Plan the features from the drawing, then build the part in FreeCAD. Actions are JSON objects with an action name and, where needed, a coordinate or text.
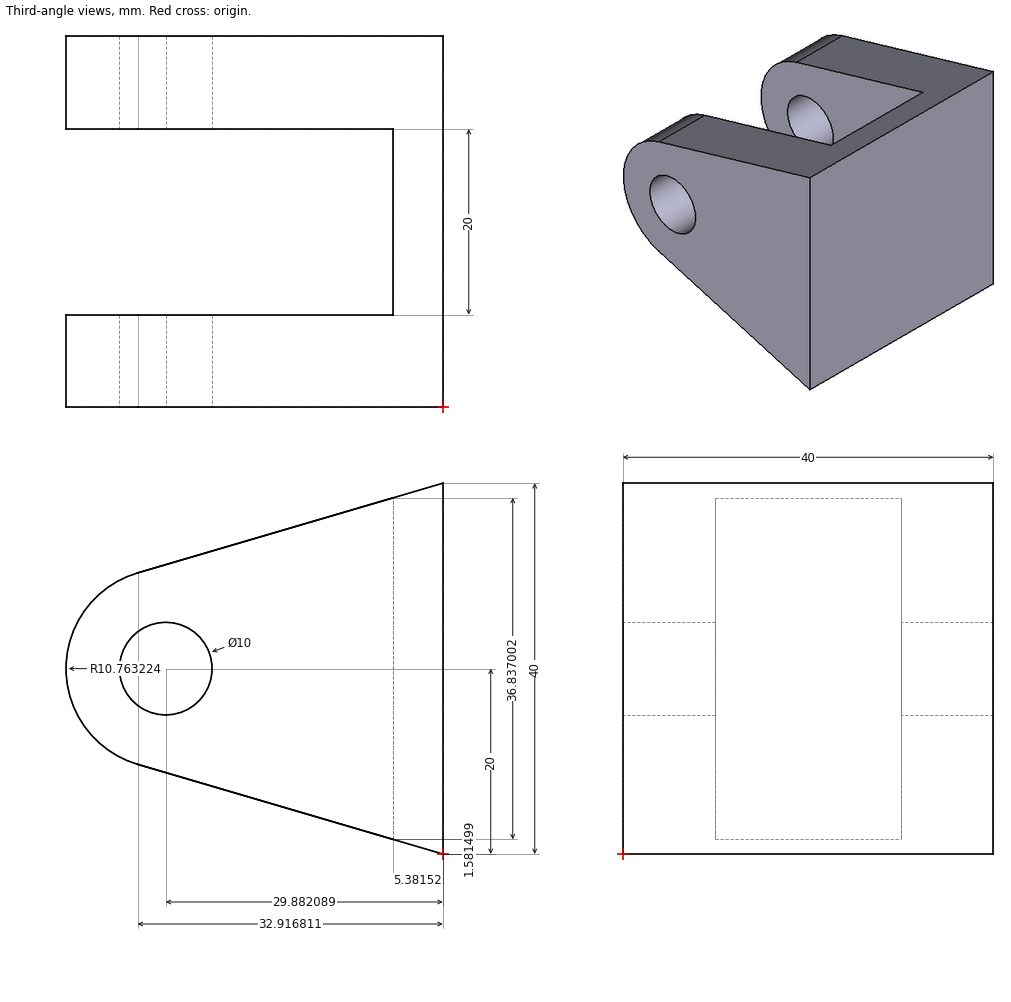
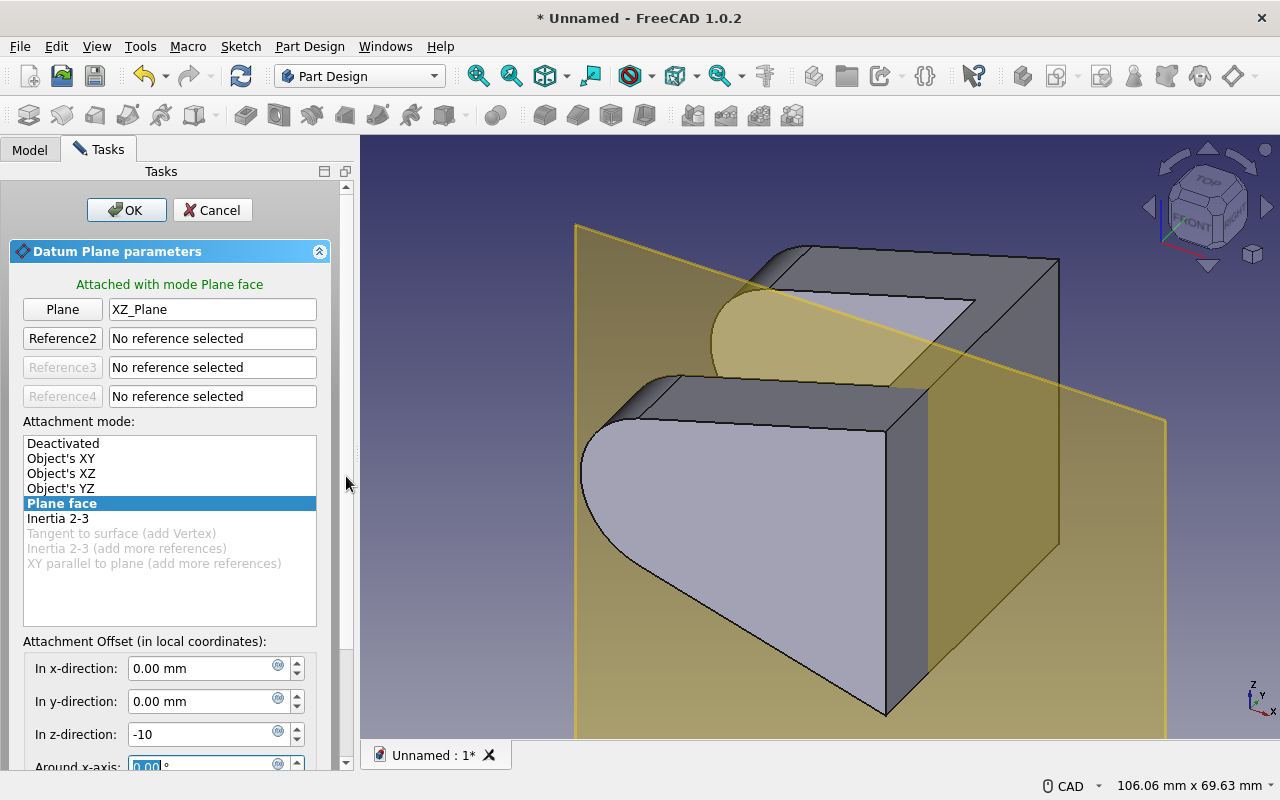
{"action": "left_click", "coordinate": [127, 210]}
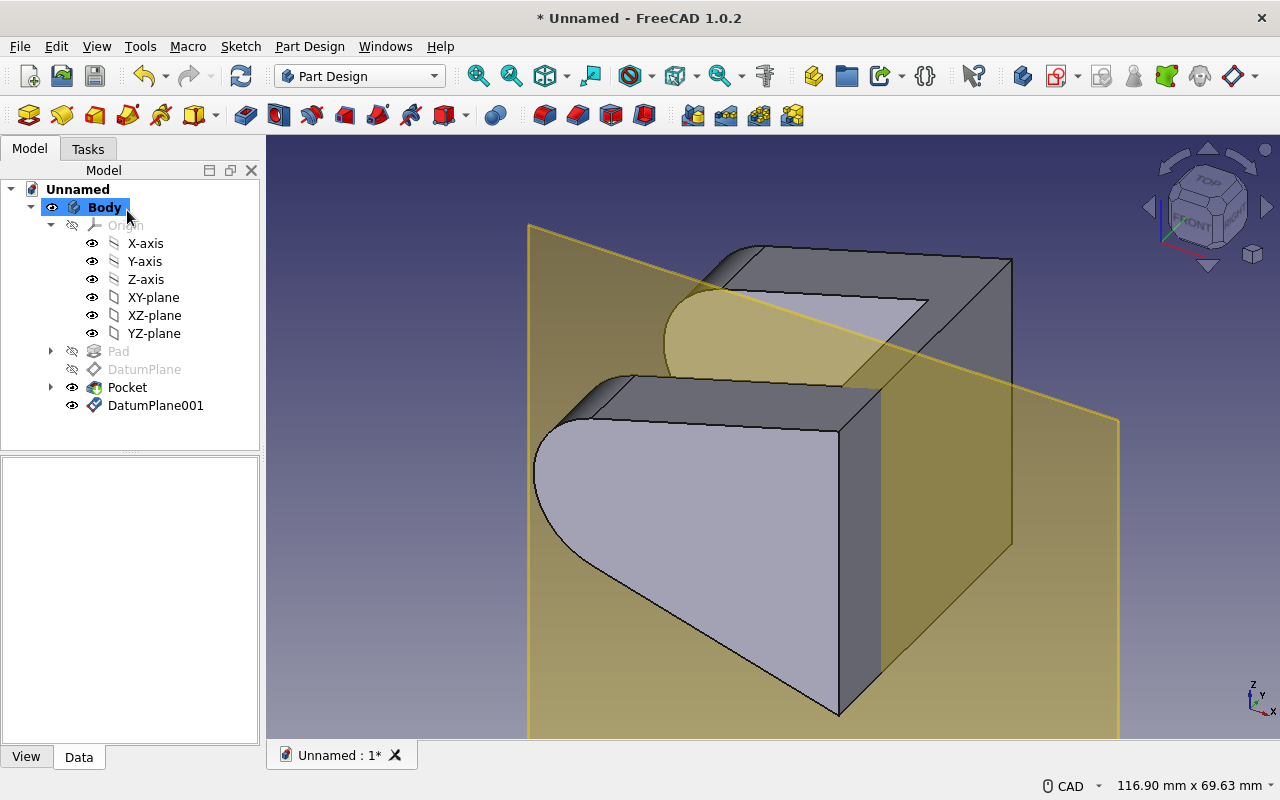
{"action": "left_click", "coordinate": [117, 405]}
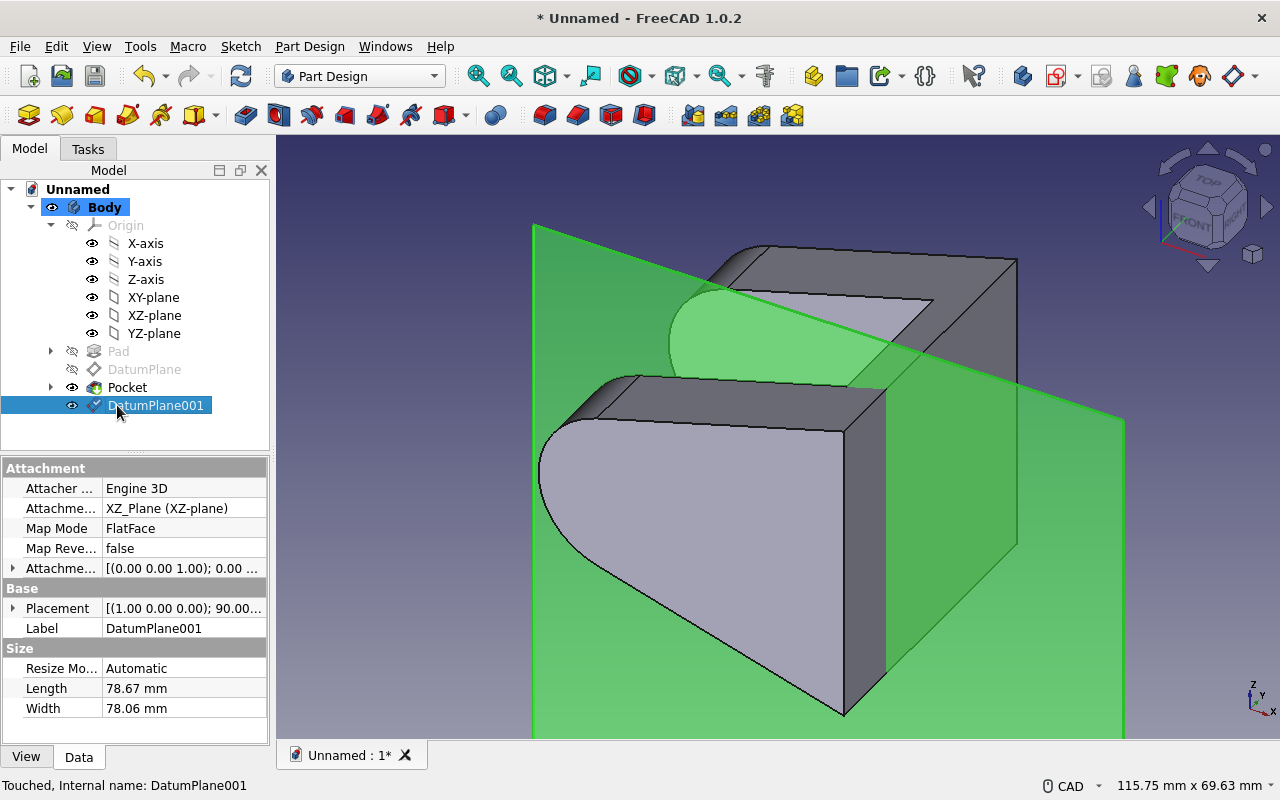
{"action": "left_click", "coordinate": [1056, 76]}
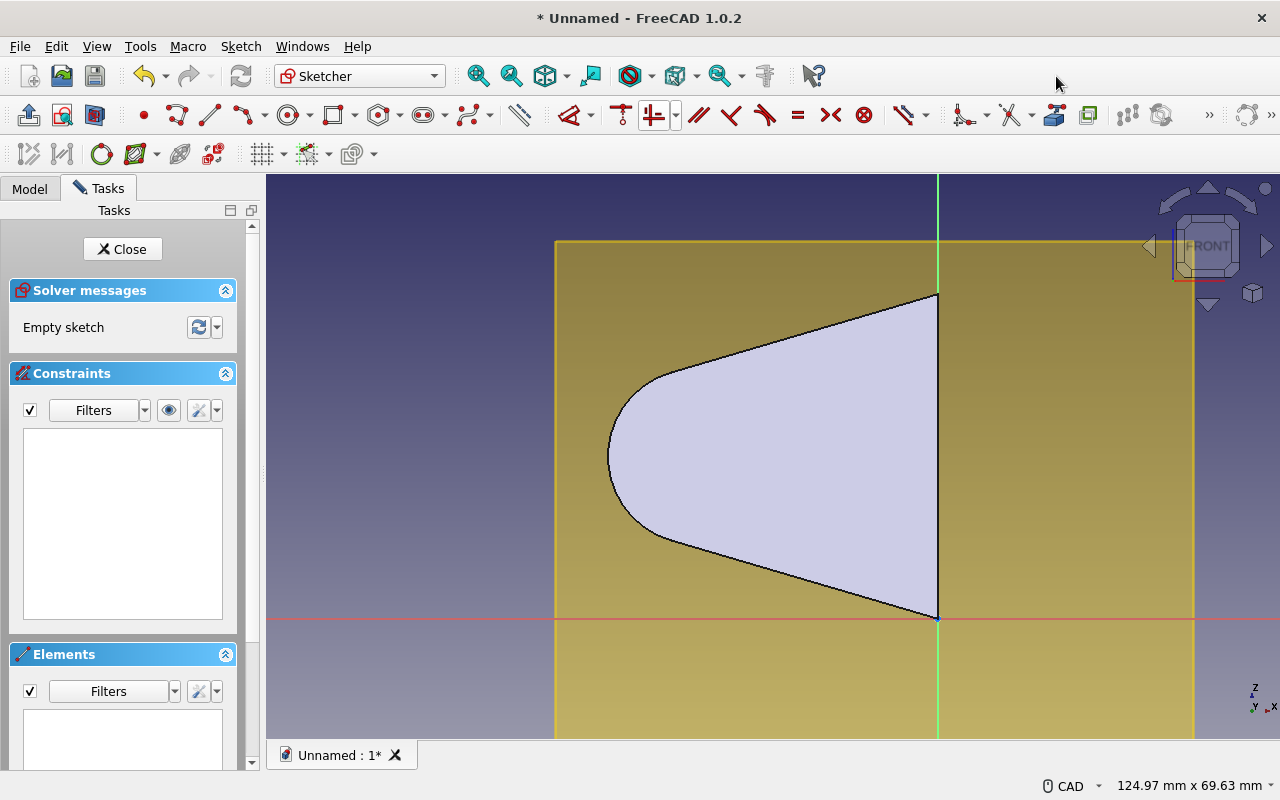
{"action": "left_click", "coordinate": [95, 116]}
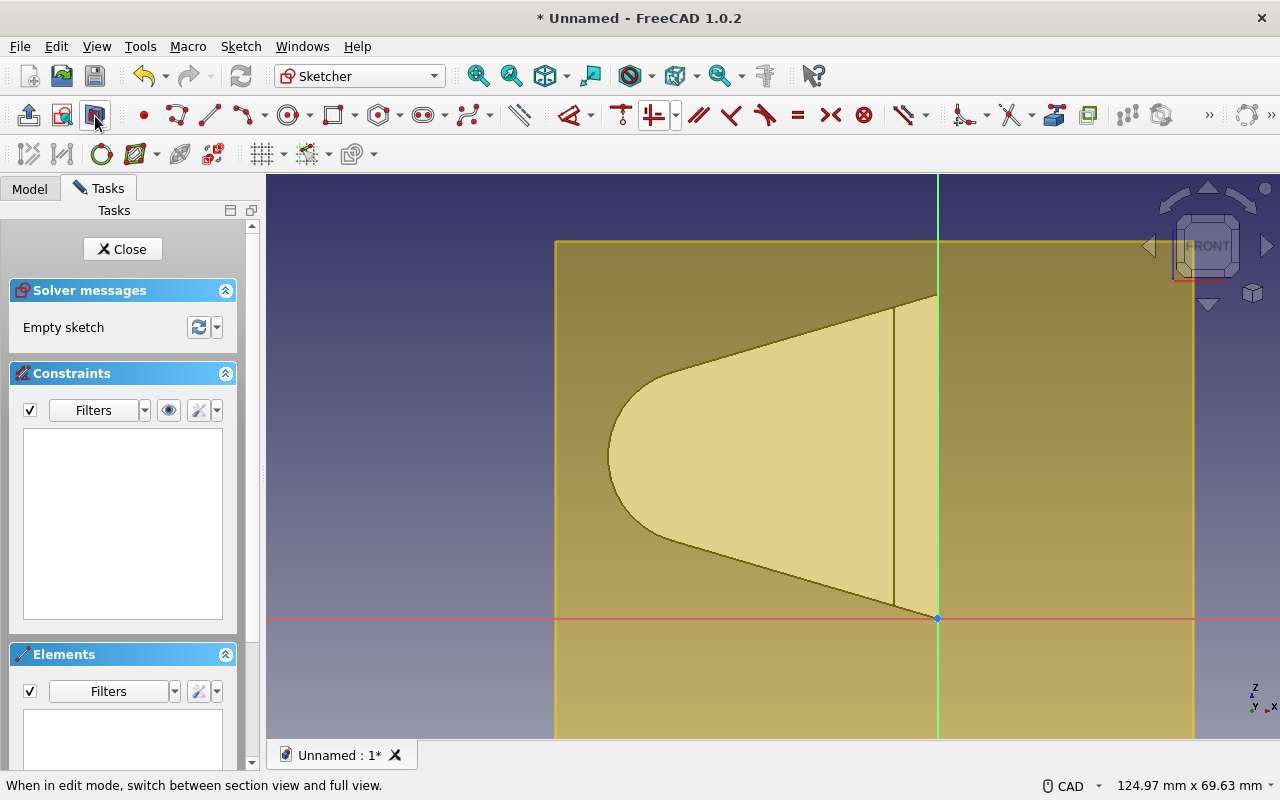
{"action": "scroll", "coordinate": [692, 457], "scroll_direction": "up", "scroll_amount": 7}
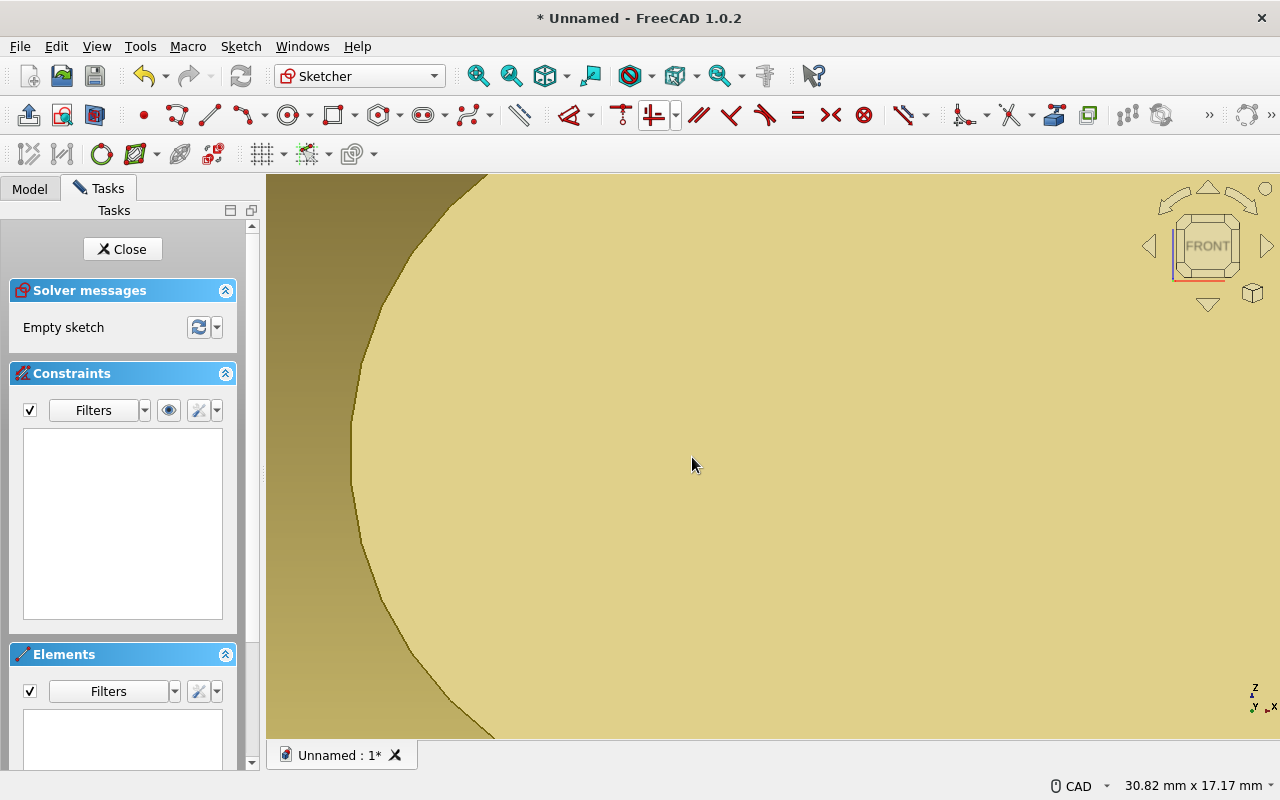
{"action": "left_click", "coordinate": [288, 116]}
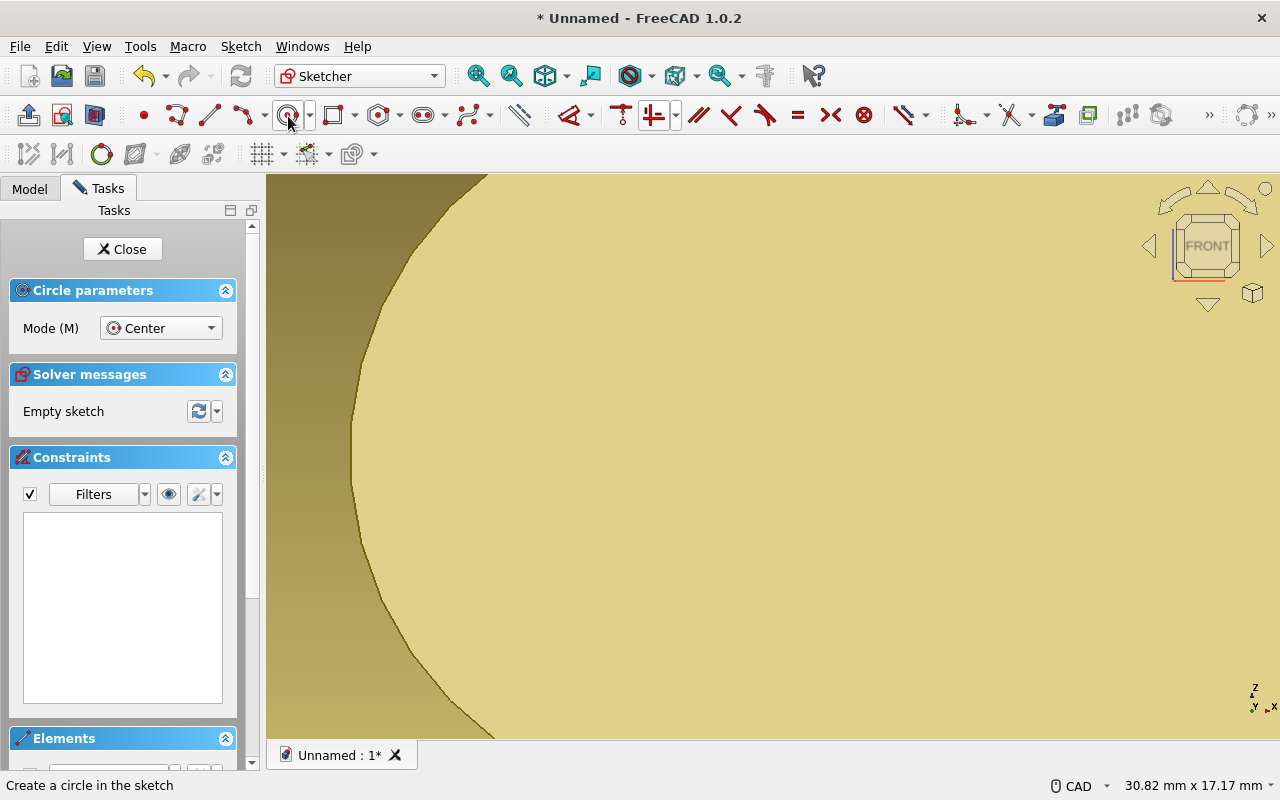
{"action": "left_click", "coordinate": [704, 453]}
{"action": "left_click", "coordinate": [820, 337]}
{"action": "key", "text": "Escape"}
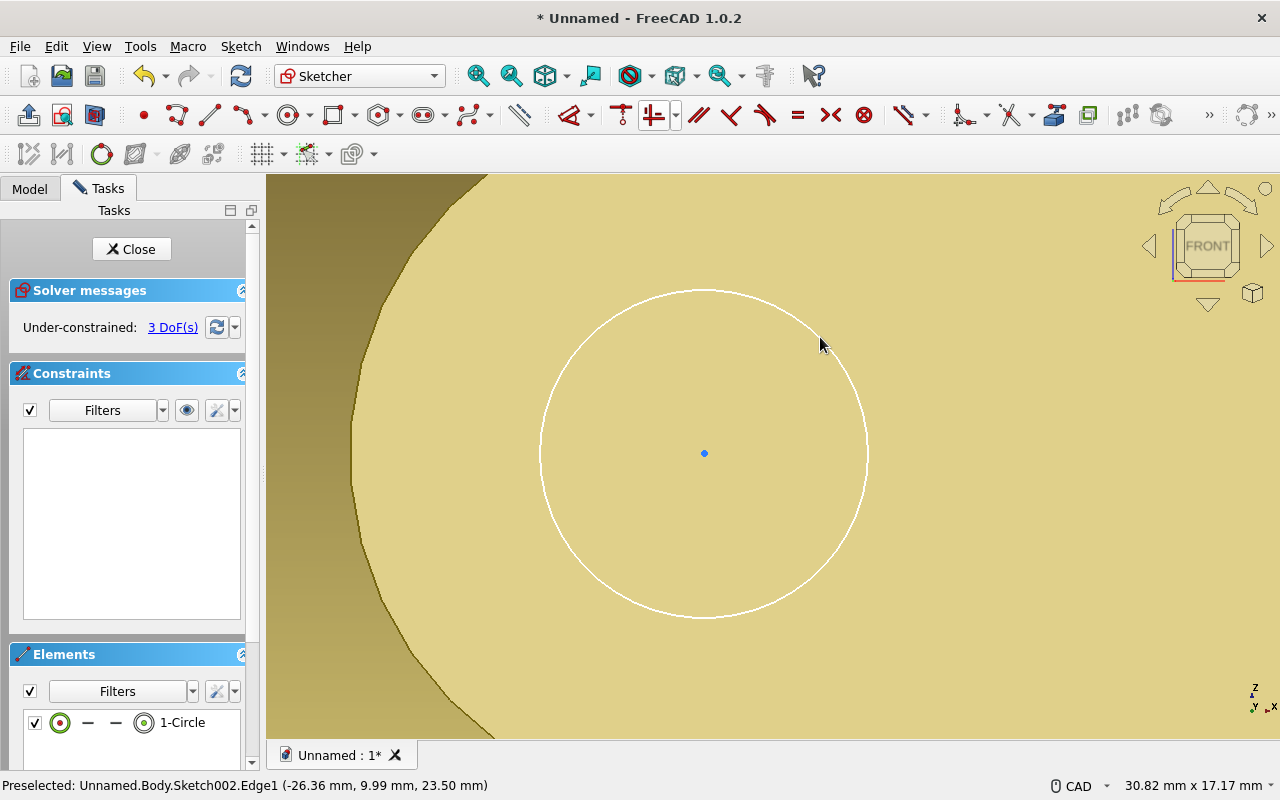
{"action": "left_click", "coordinate": [568, 116]}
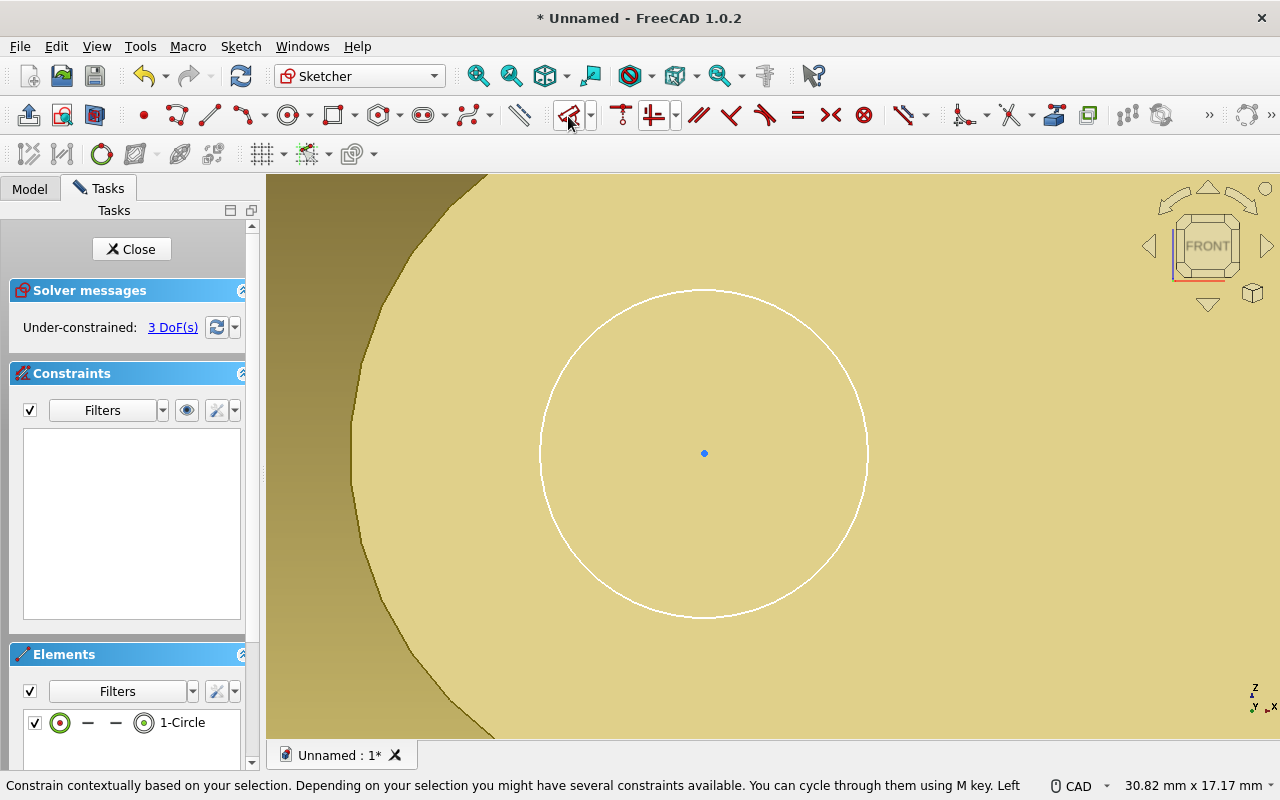
{"action": "left_click", "coordinate": [820, 338]}
{"action": "left_click", "coordinate": [843, 315]}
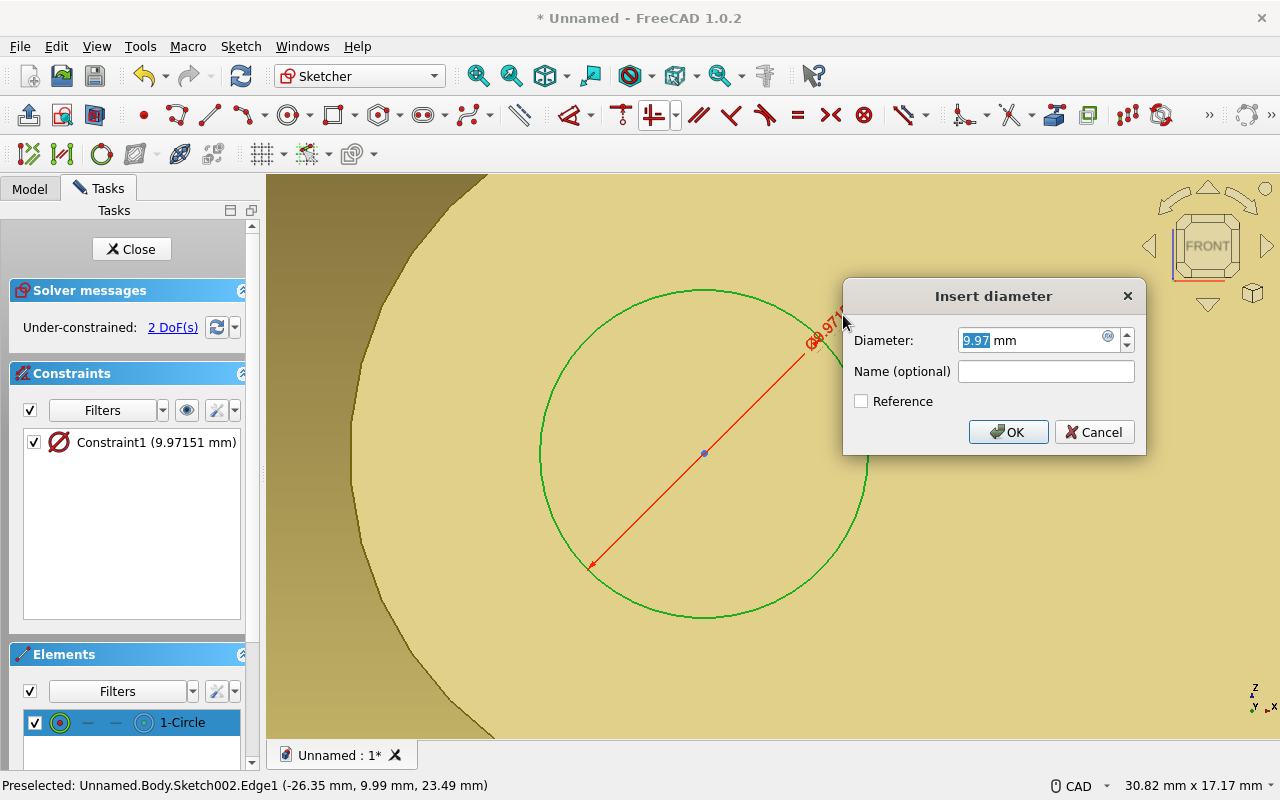
{"action": "type", "text": "10"}
{"action": "key", "text": "Return"}